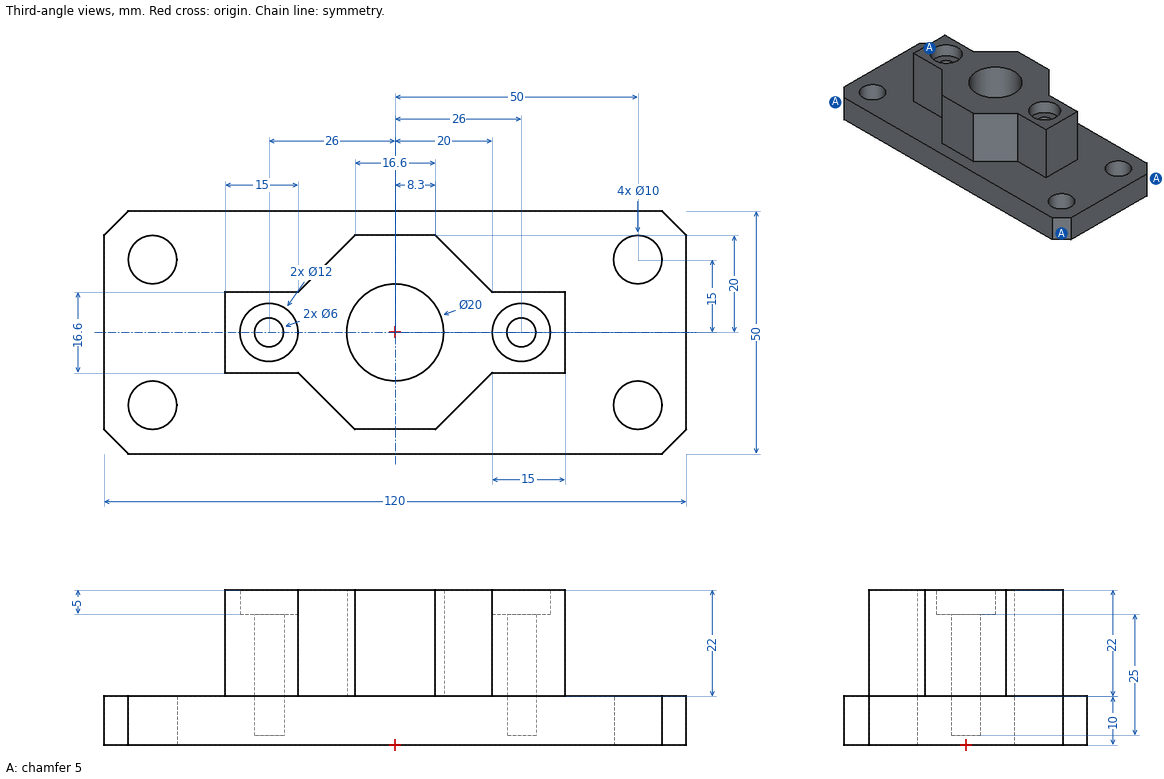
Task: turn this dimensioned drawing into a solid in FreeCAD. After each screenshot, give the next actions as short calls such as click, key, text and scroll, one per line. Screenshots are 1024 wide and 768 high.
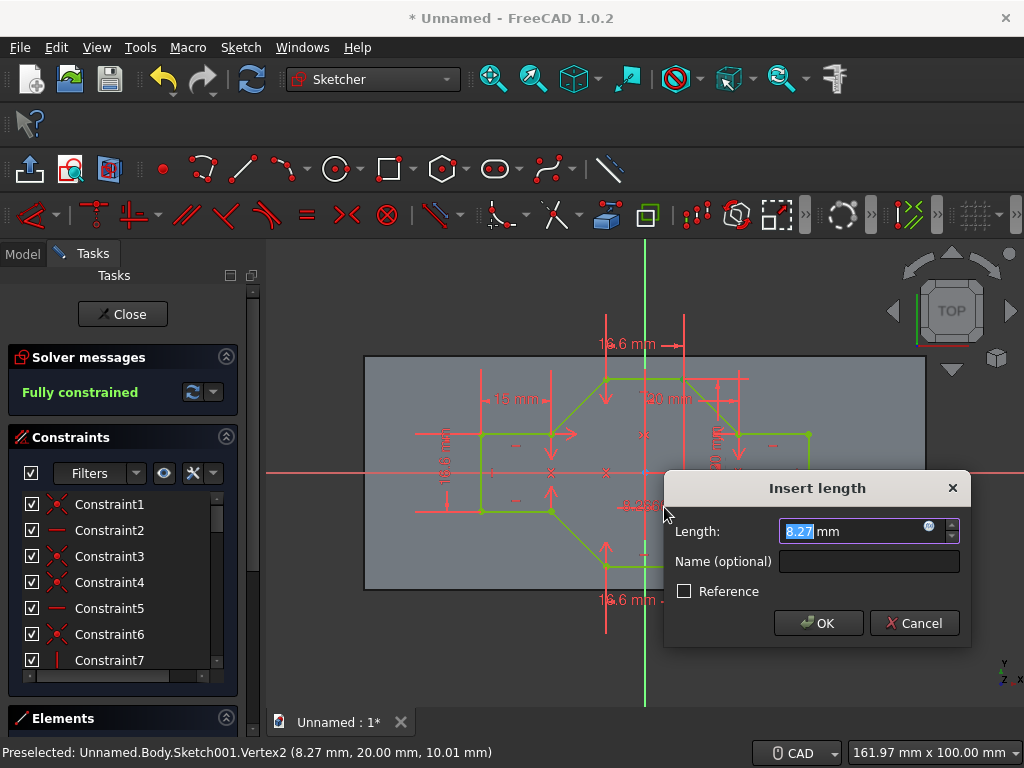
text(8.3)
key(Return)
key(Escape)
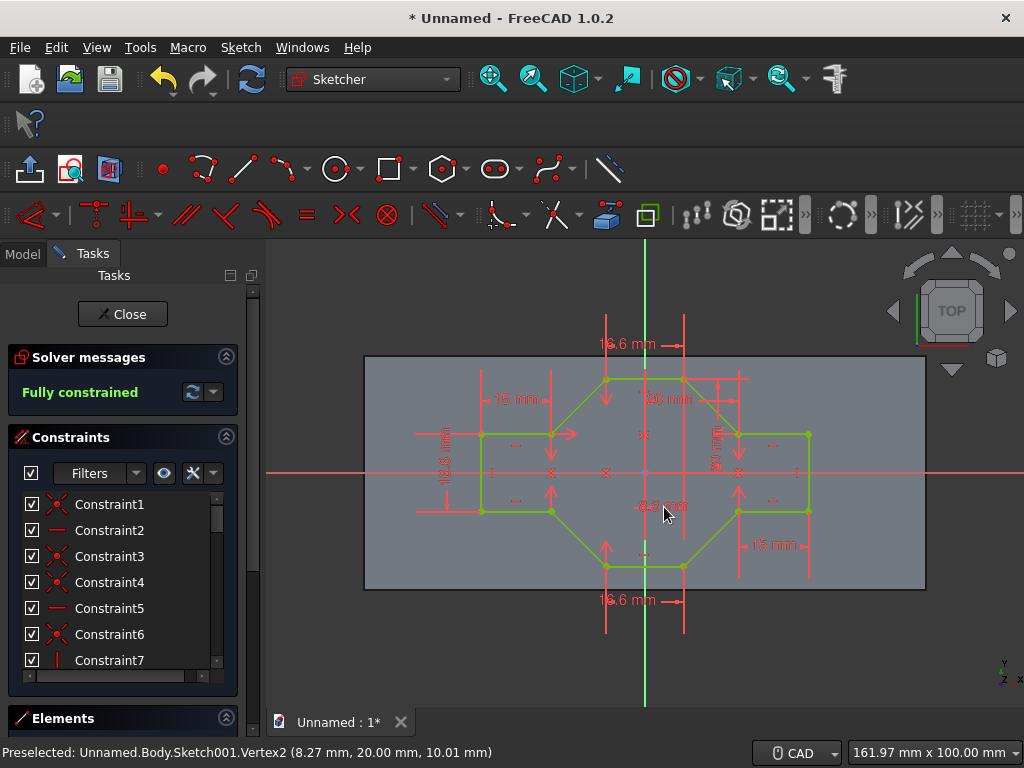
click(123, 314)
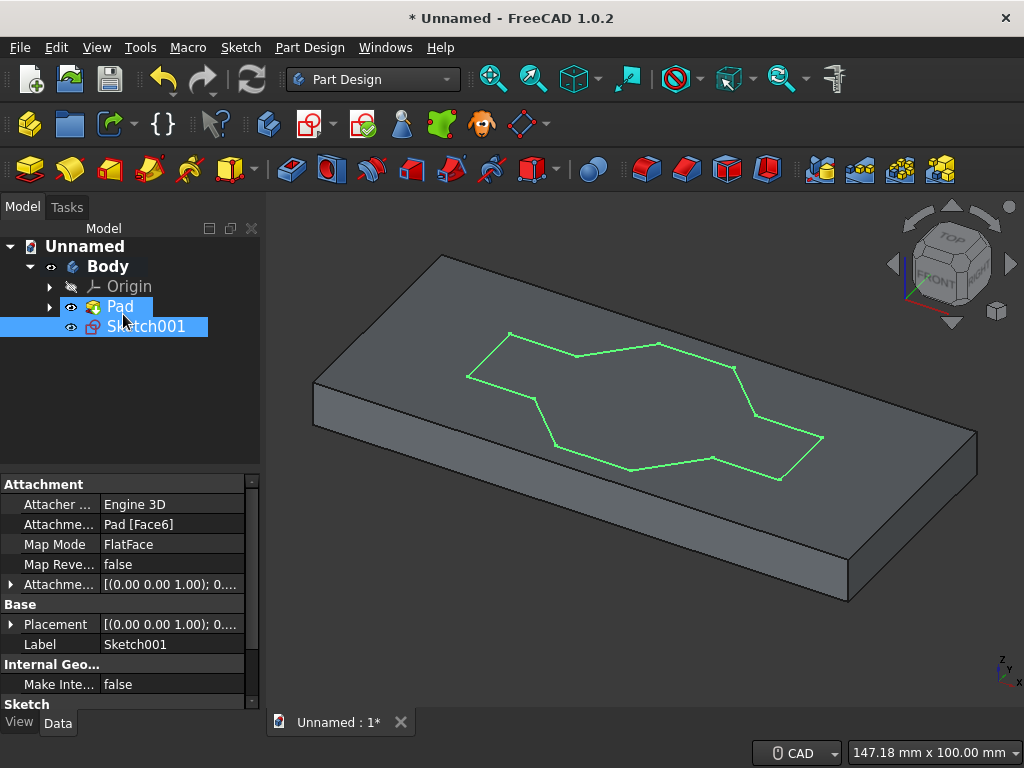
click(30, 170)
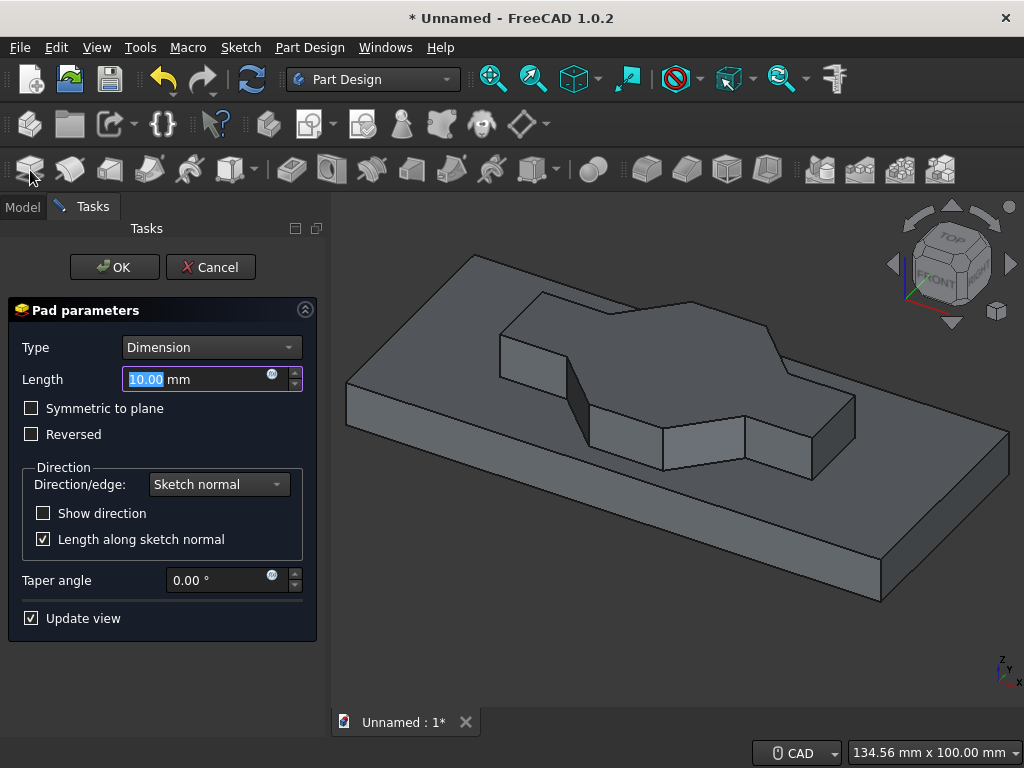
text(22)
key(Tab)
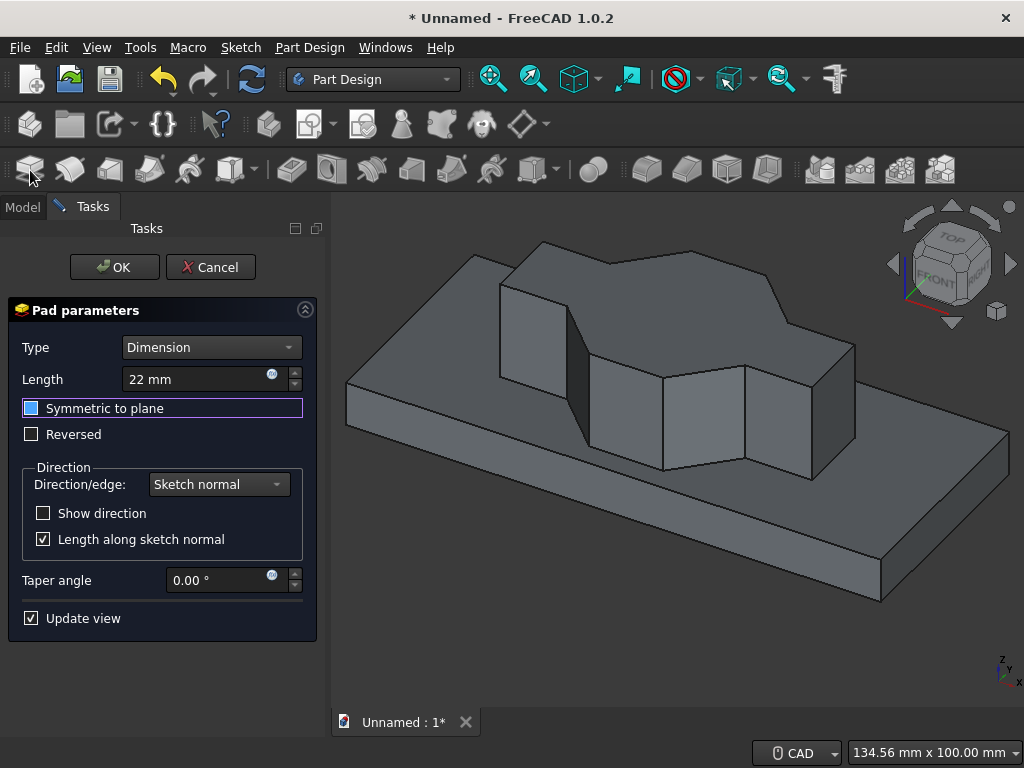
click(115, 267)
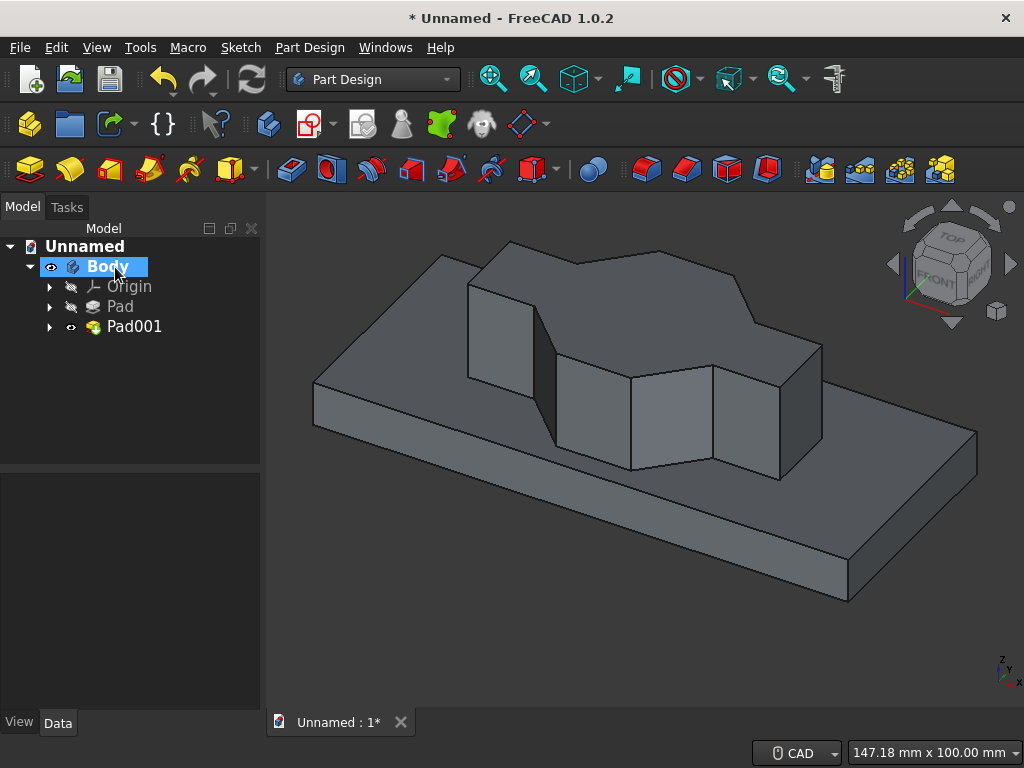
click(494, 80)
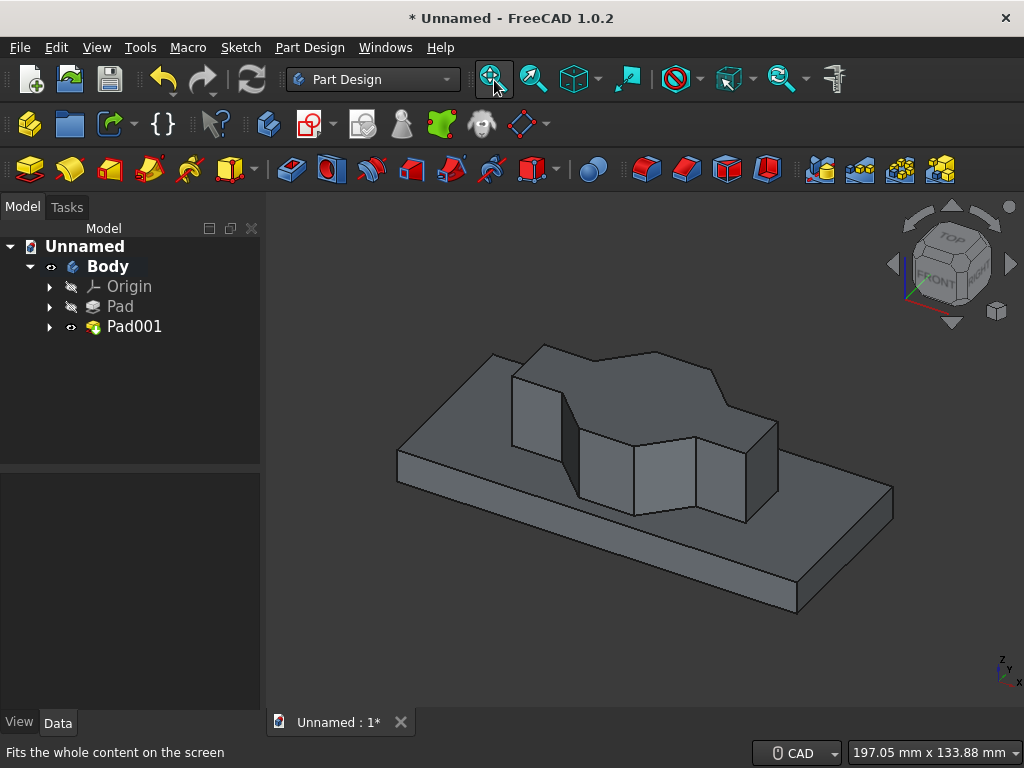
click(645, 398)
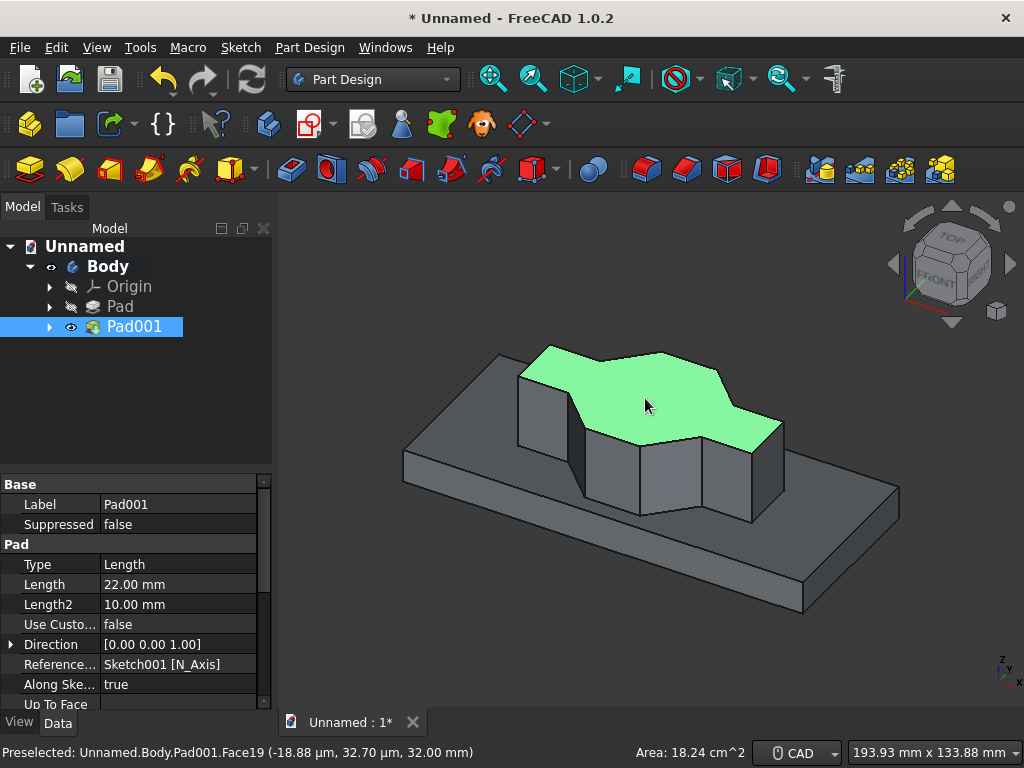
click(310, 124)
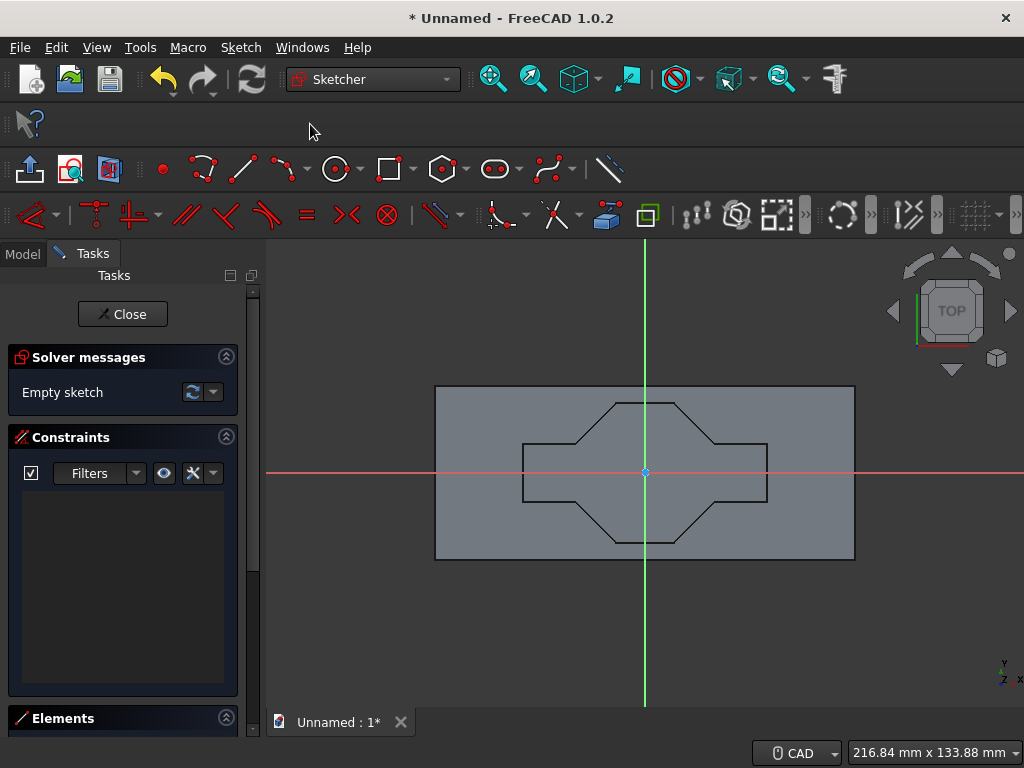
scroll(667, 473, up, 7)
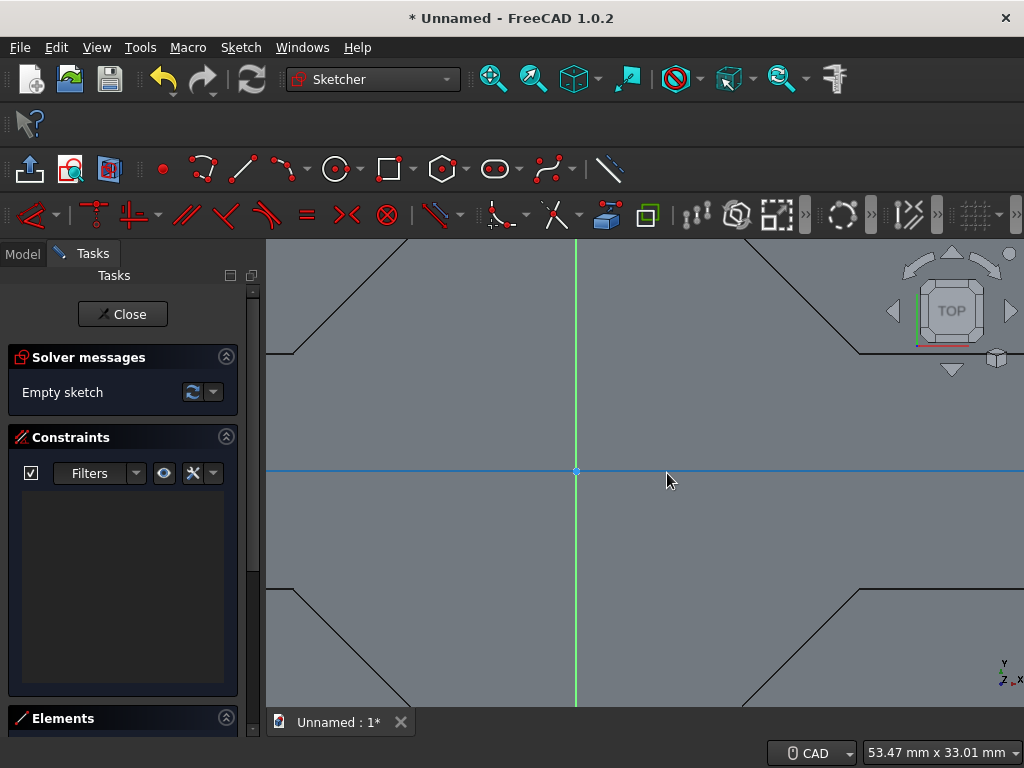
click(336, 170)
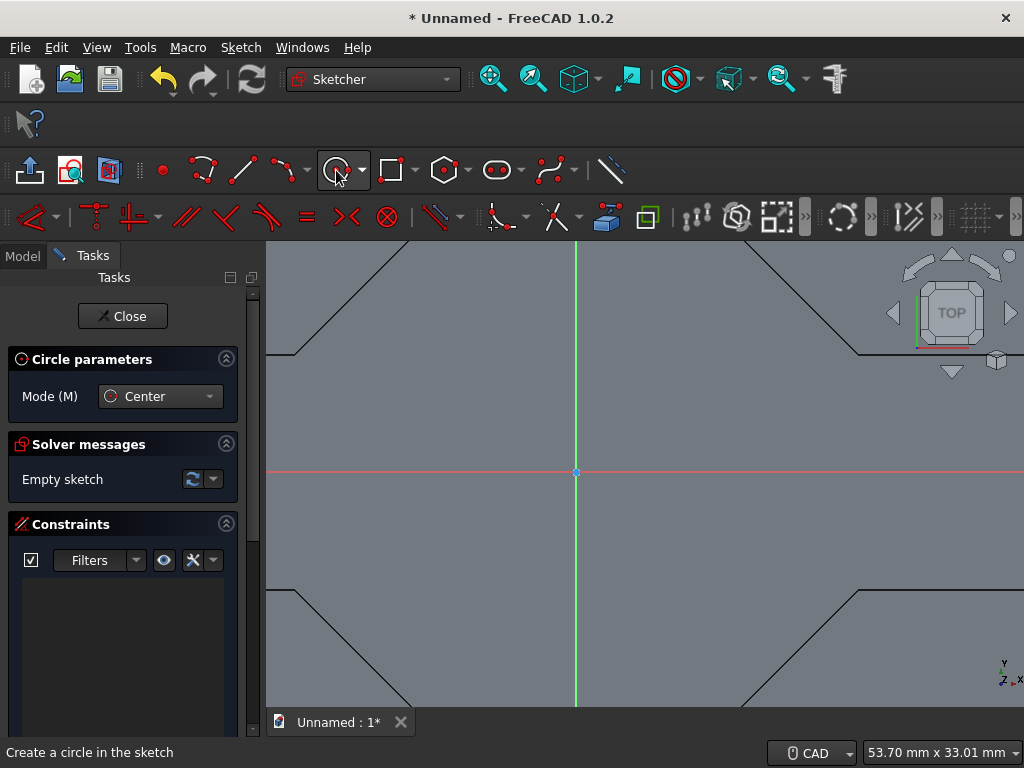
click(576, 472)
click(676, 373)
key(Escape)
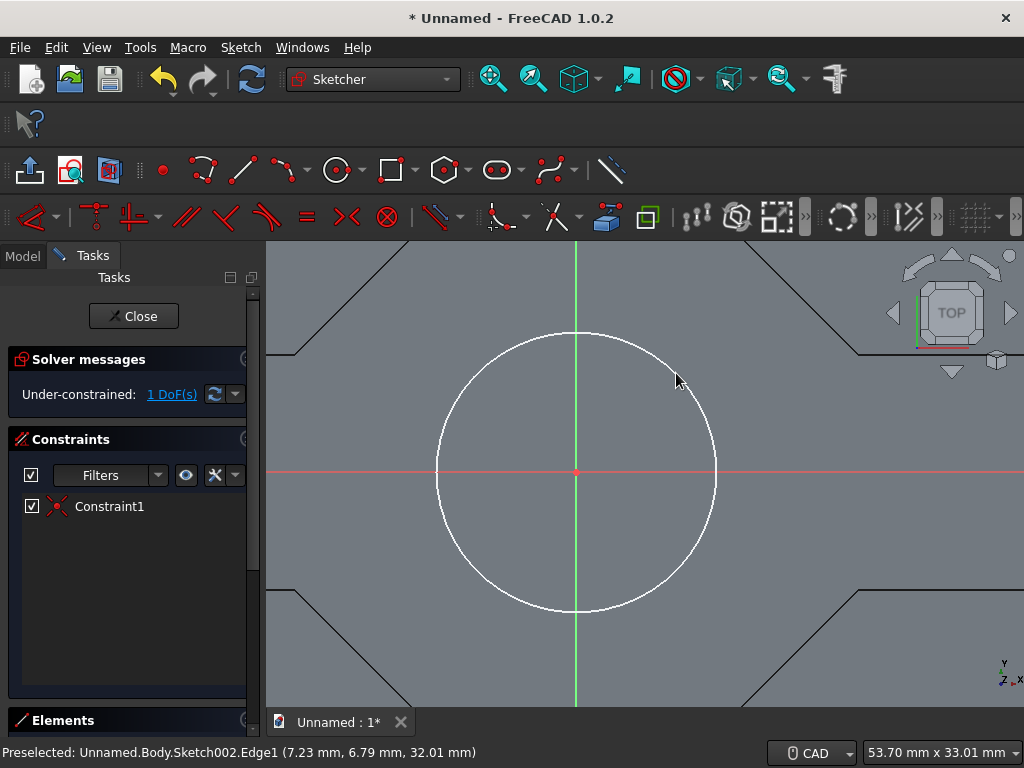
click(32, 218)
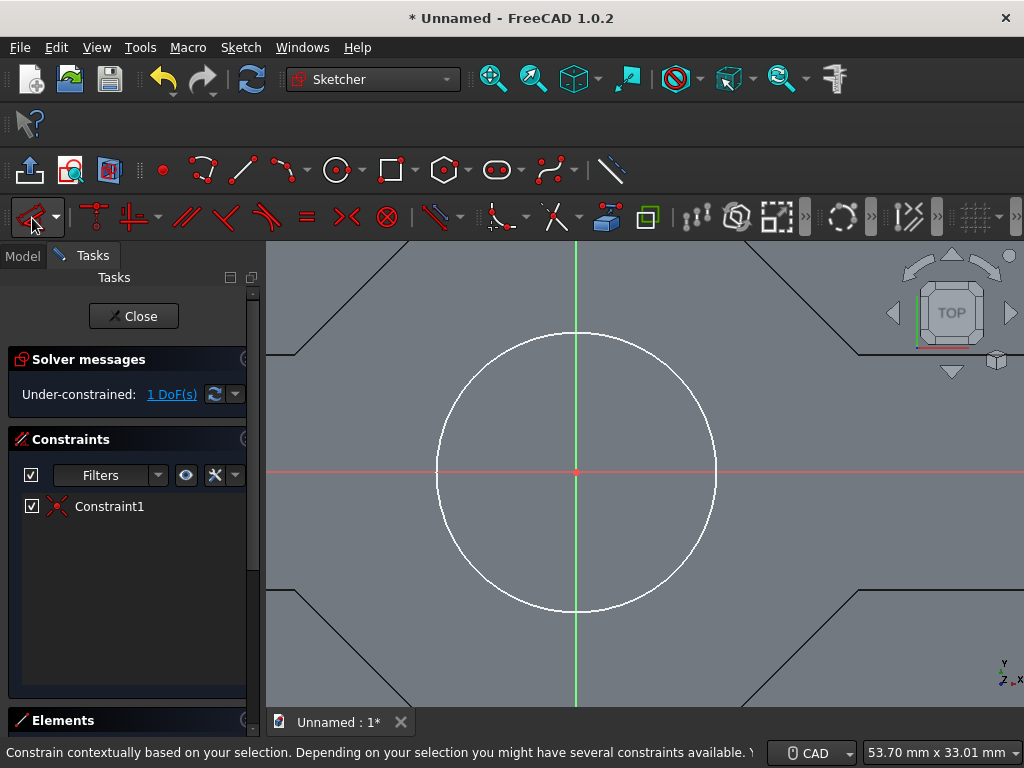
click(675, 373)
click(698, 350)